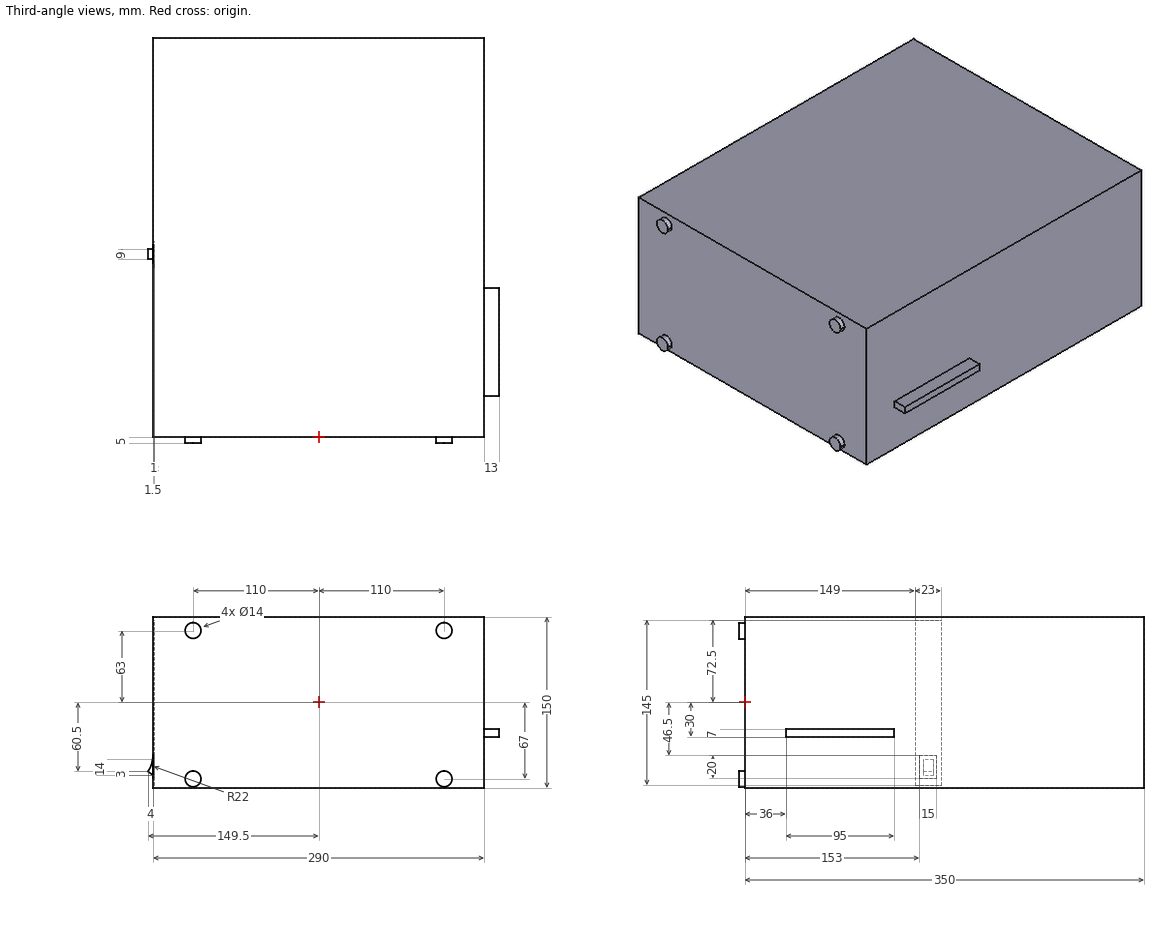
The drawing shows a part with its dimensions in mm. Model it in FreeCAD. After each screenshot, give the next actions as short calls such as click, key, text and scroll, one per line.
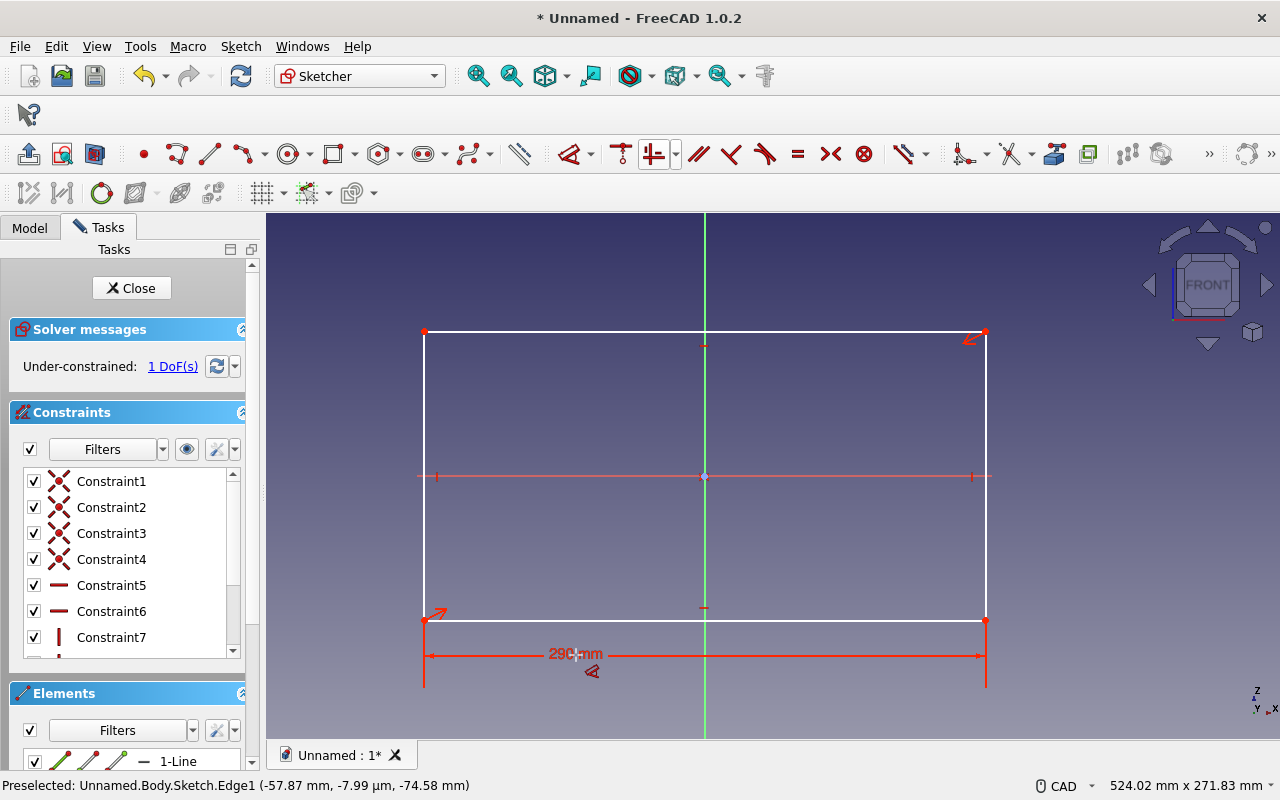
click(986, 534)
click(1020, 410)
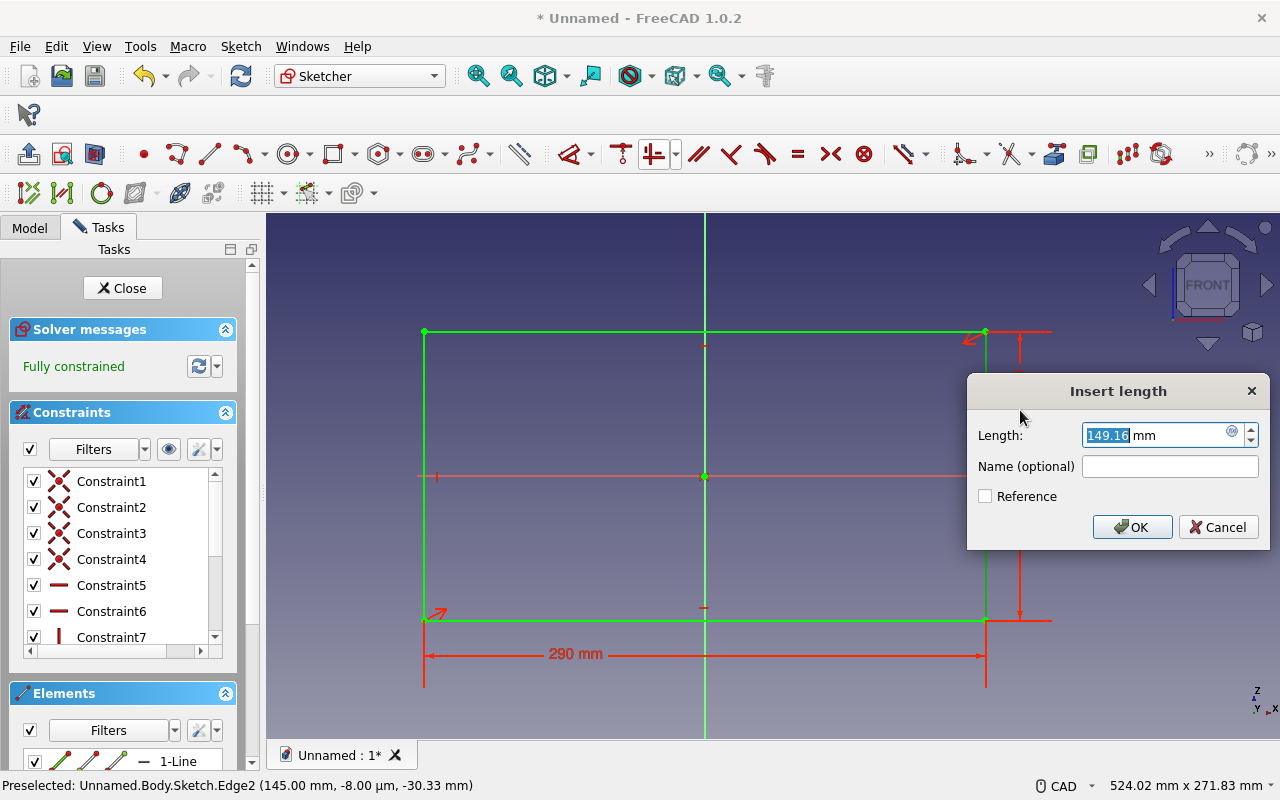
text(150)
key(Return)
key(Escape)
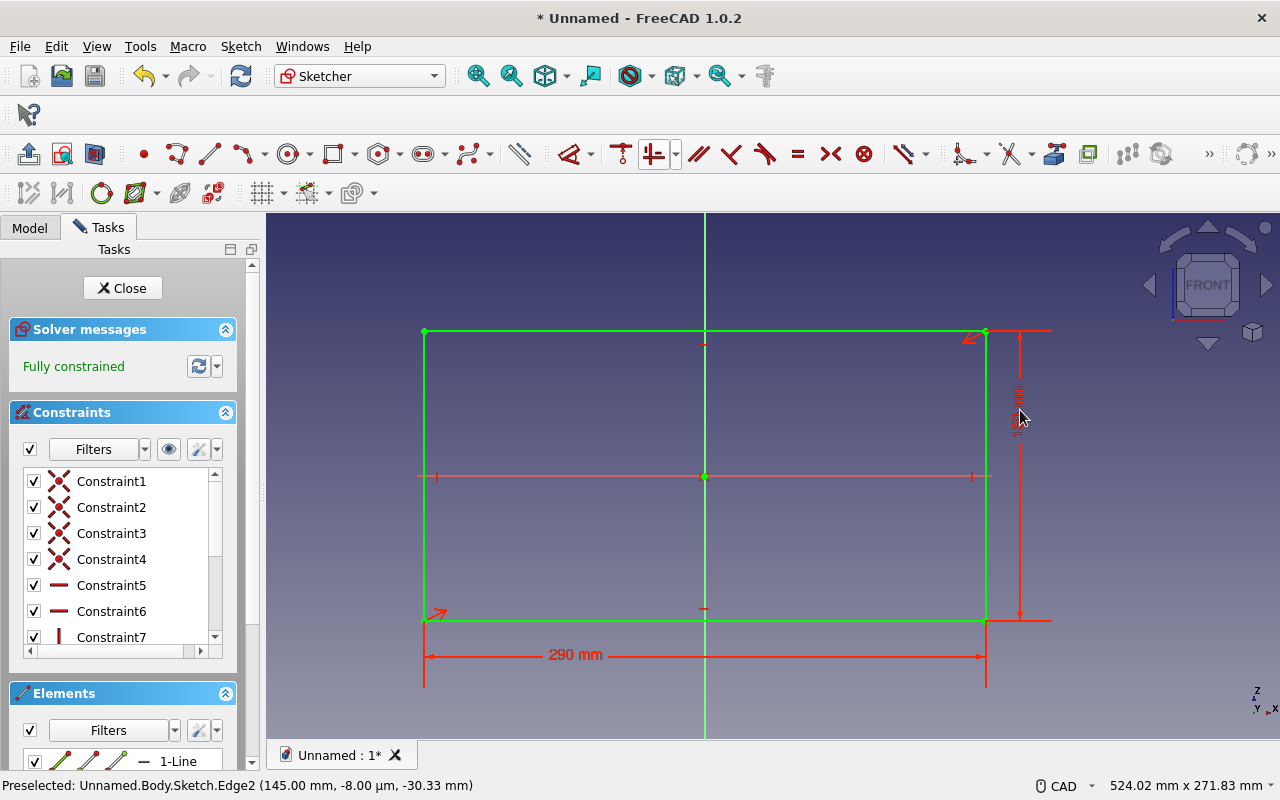
click(123, 288)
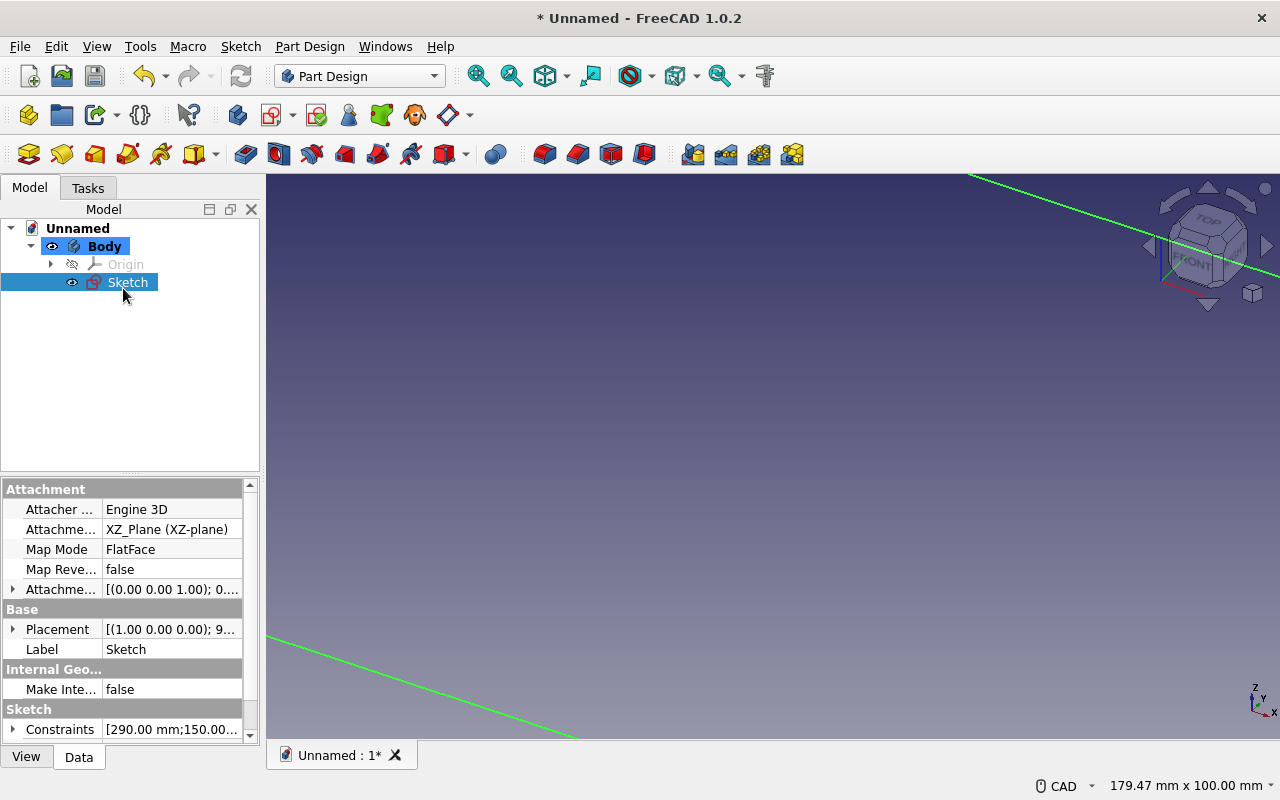
click(29, 154)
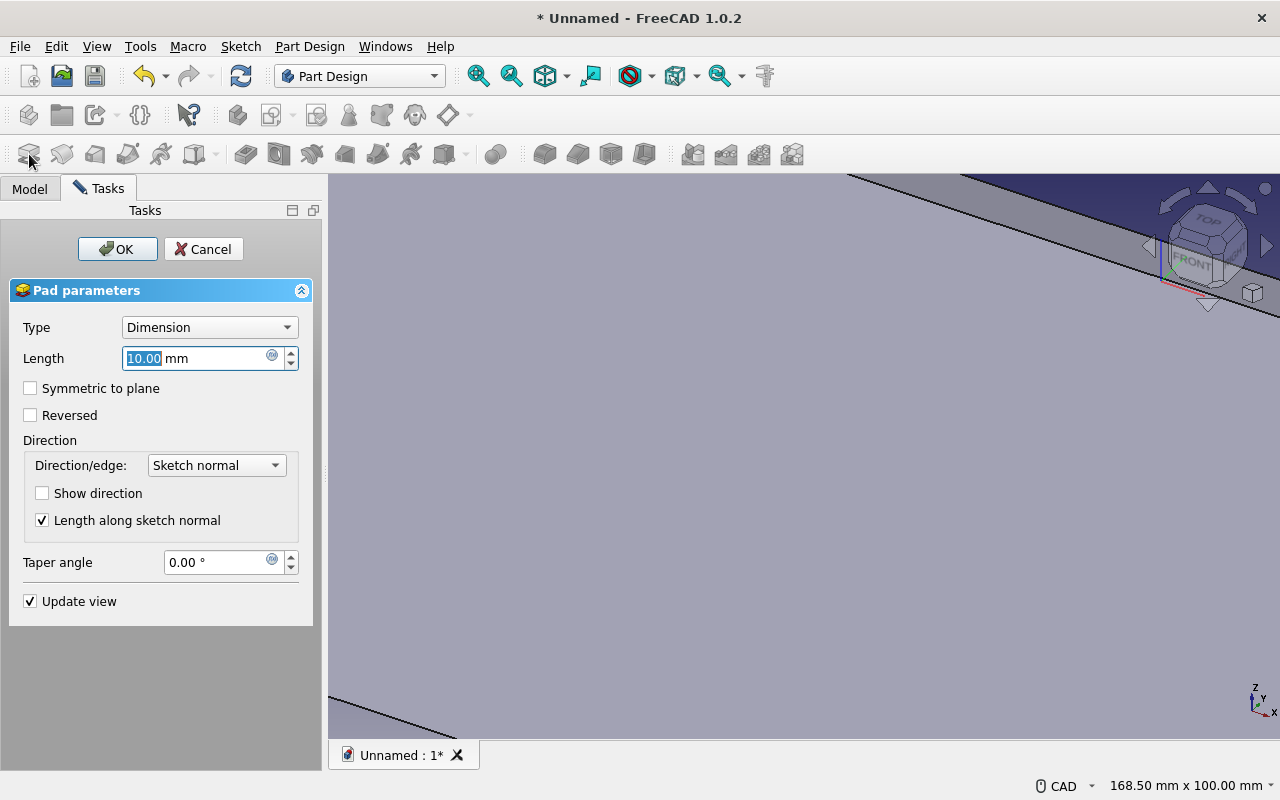
text(350)
key(Tab)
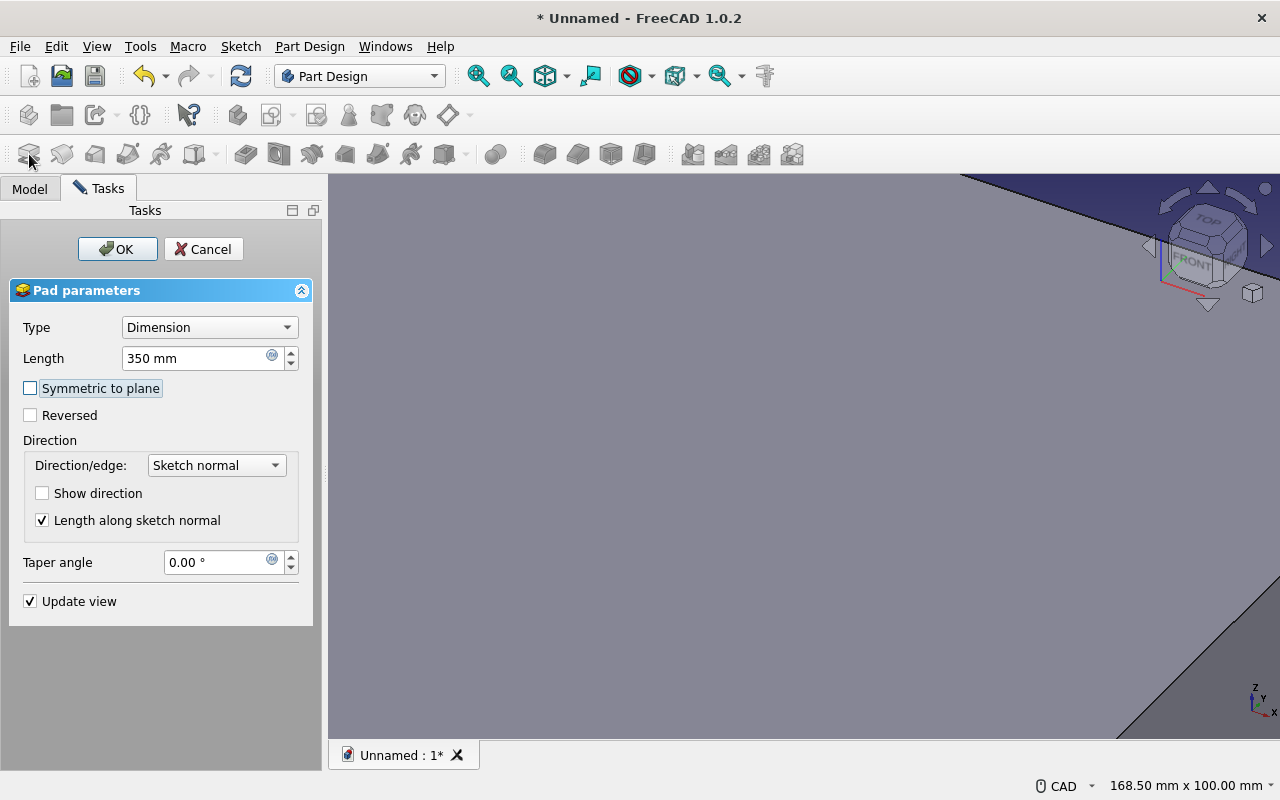
click(31, 415)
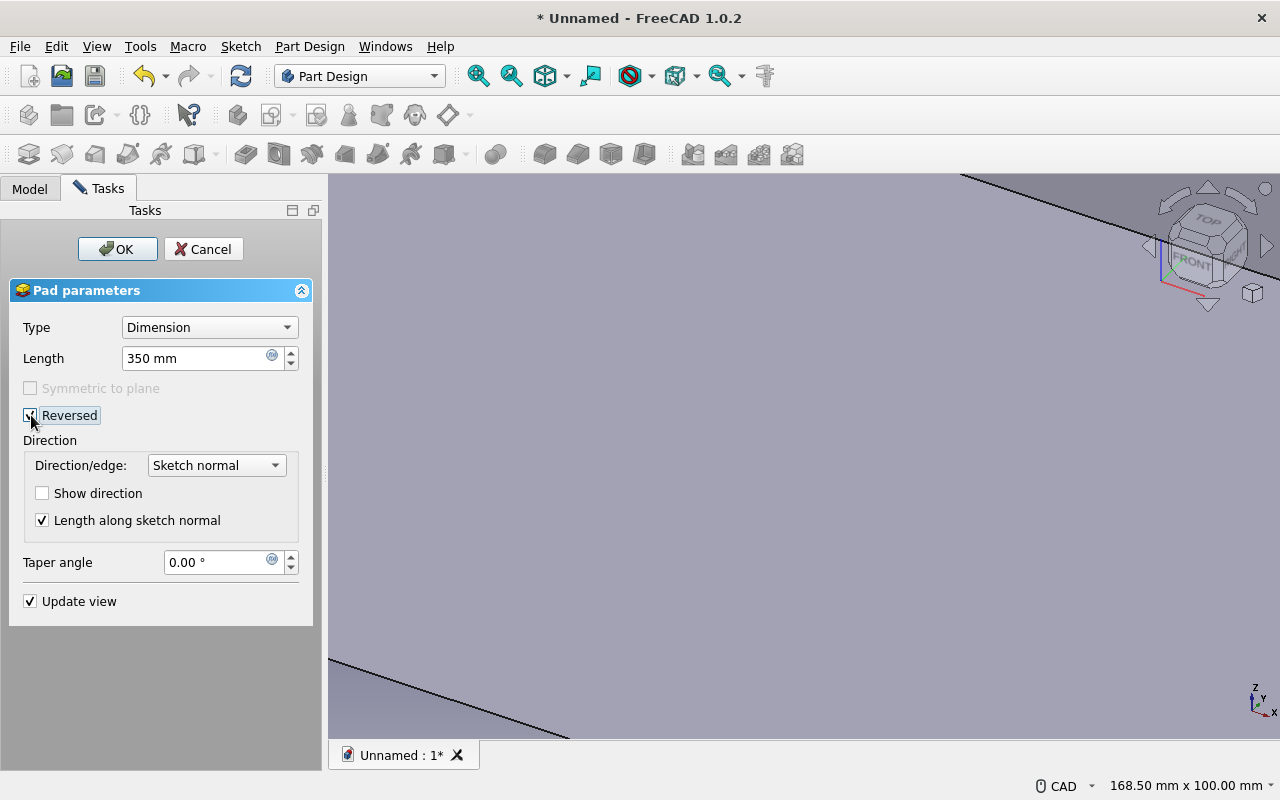
click(118, 249)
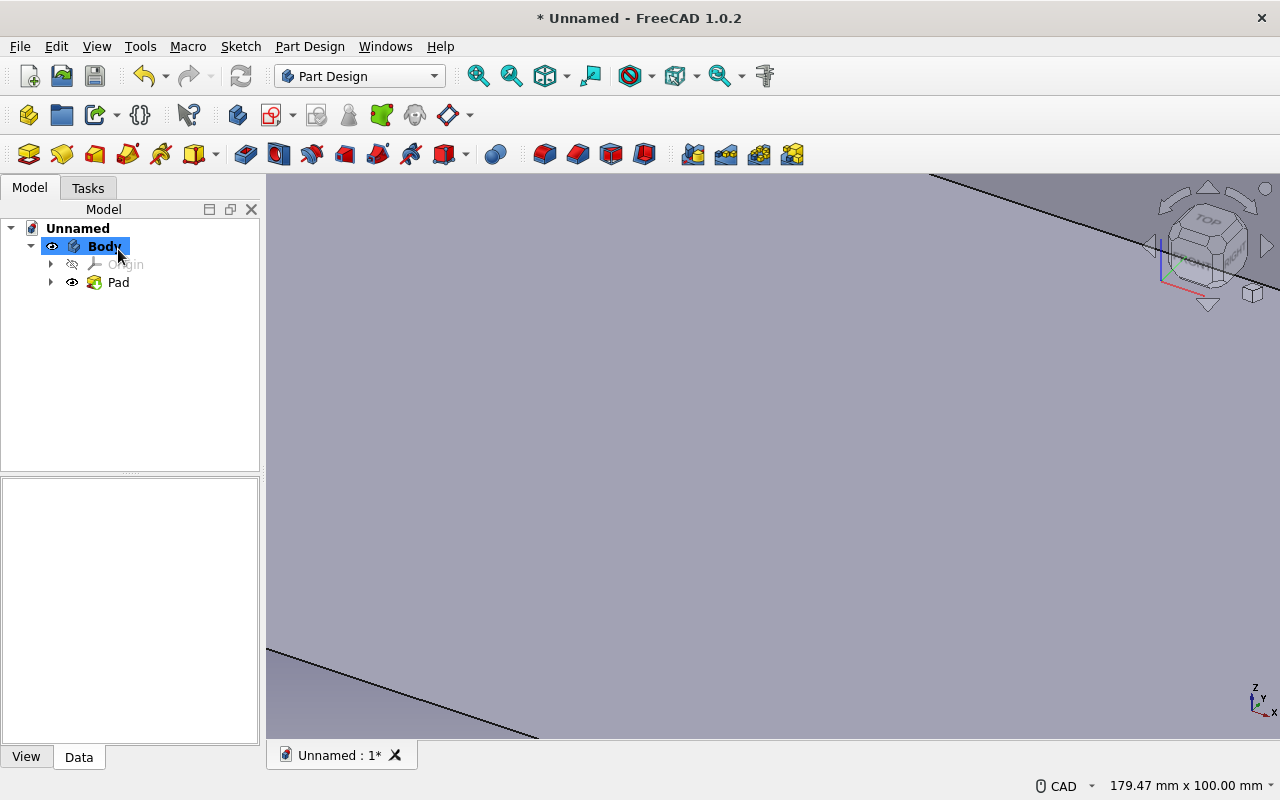
click(479, 76)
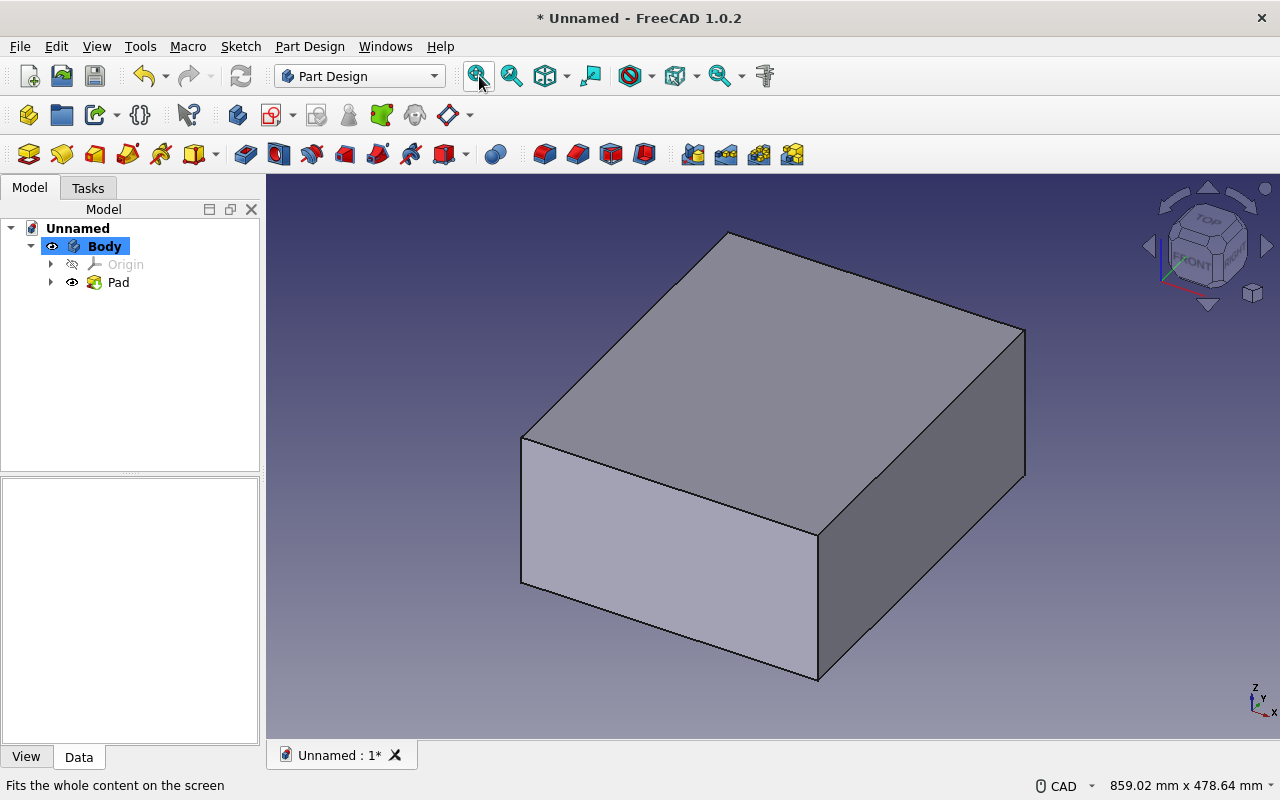
click(270, 116)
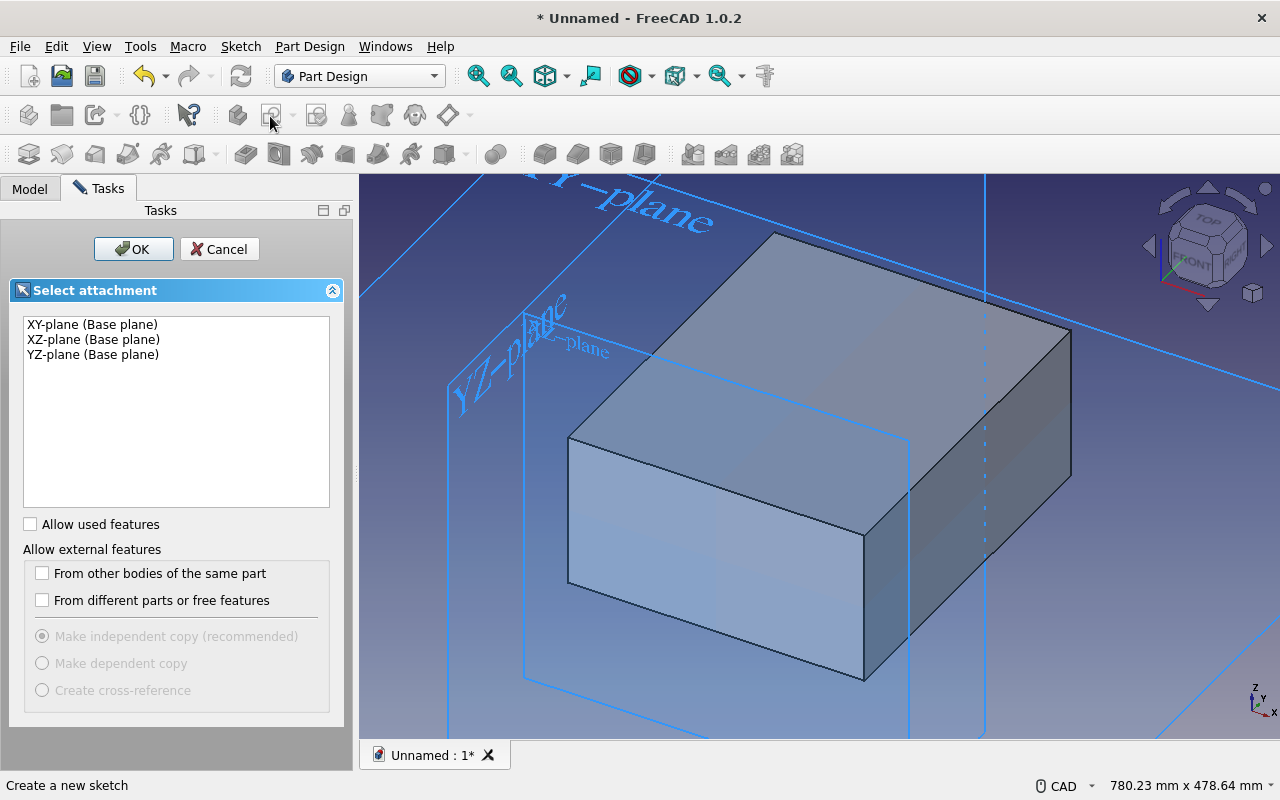
click(84, 340)